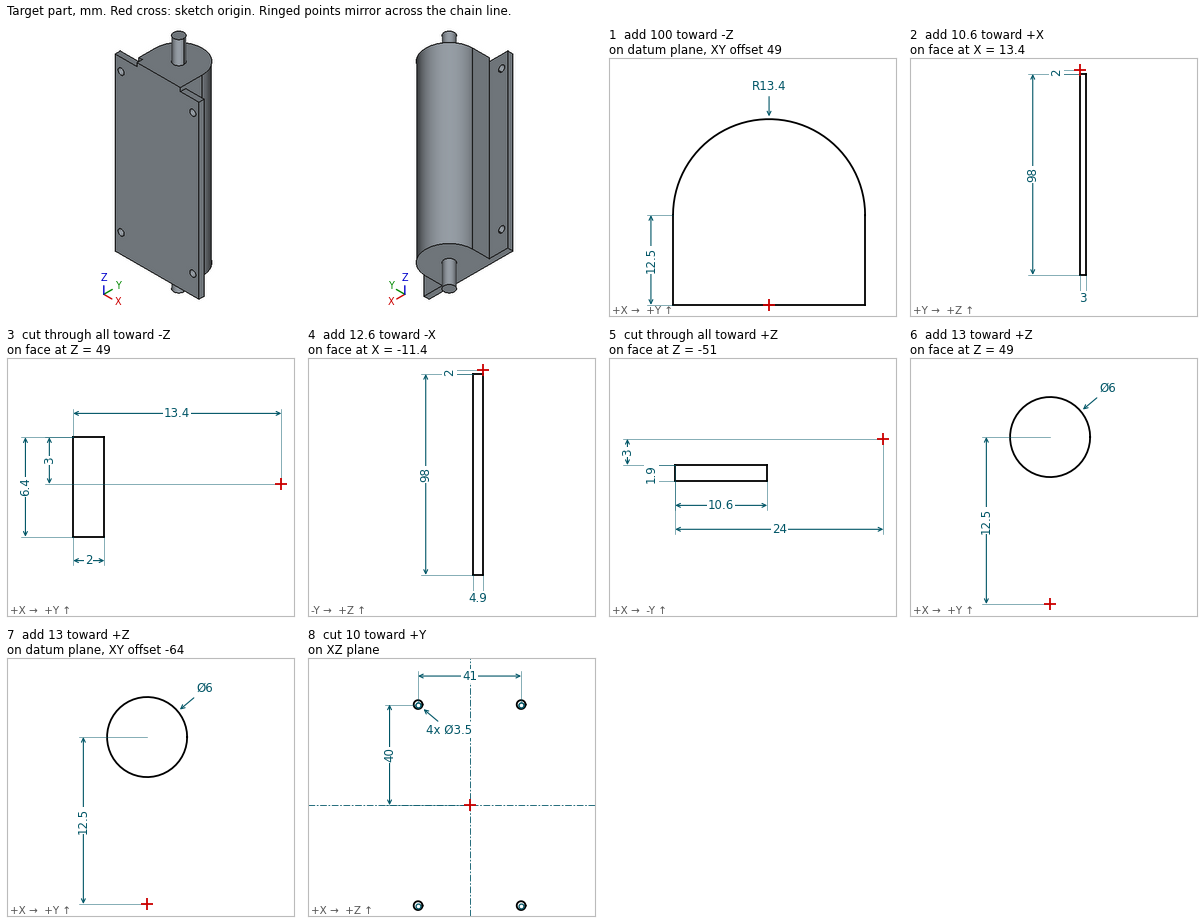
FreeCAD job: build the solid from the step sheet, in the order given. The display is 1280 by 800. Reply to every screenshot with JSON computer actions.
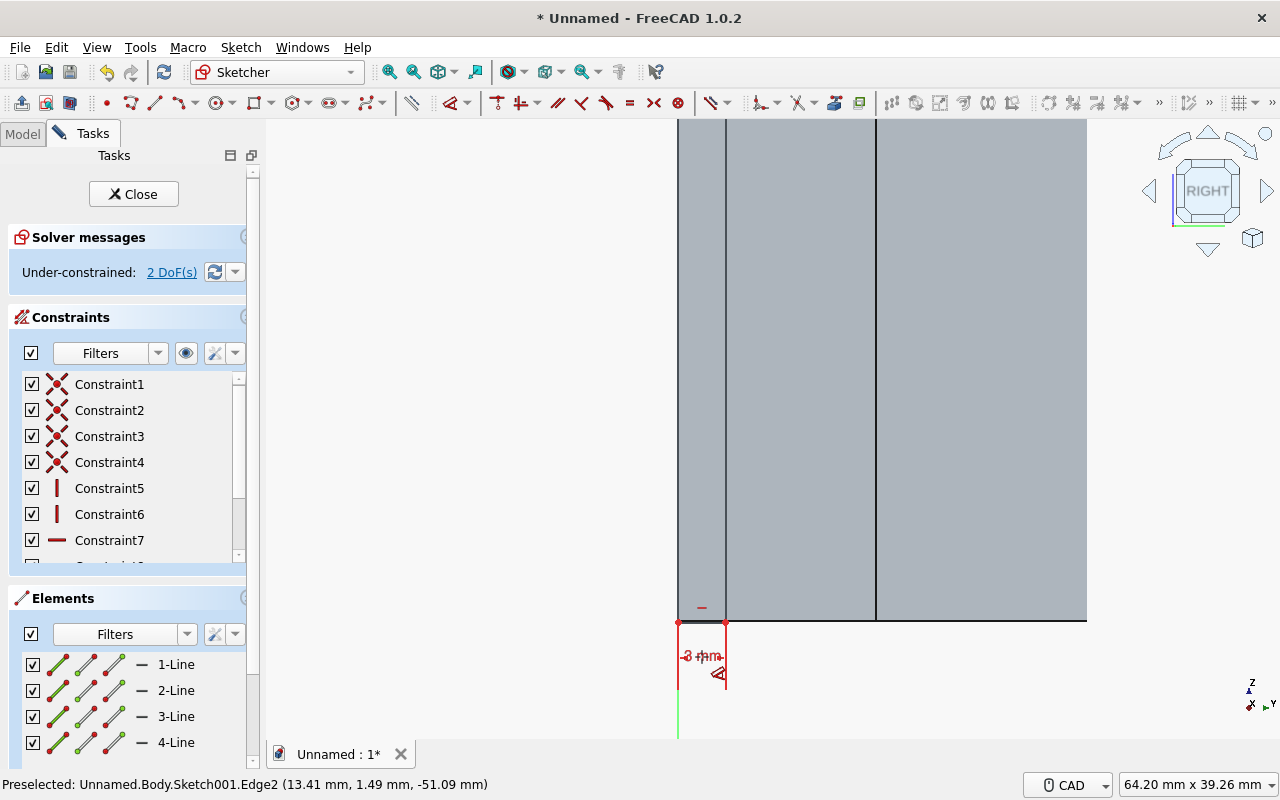
{"action": "scroll", "coordinate": [705, 625], "scroll_direction": "down", "scroll_amount": 7}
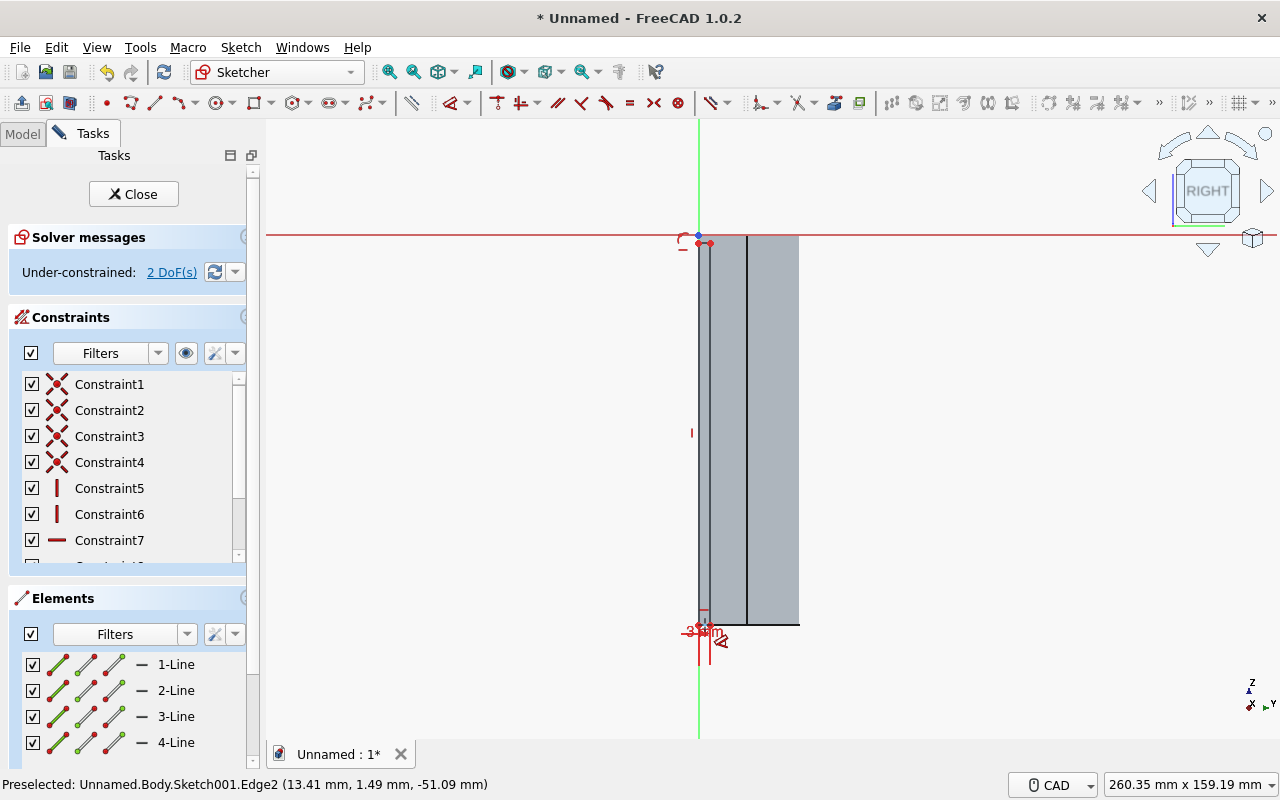
{"action": "left_click", "coordinate": [699, 511]}
{"action": "left_click", "coordinate": [665, 434]}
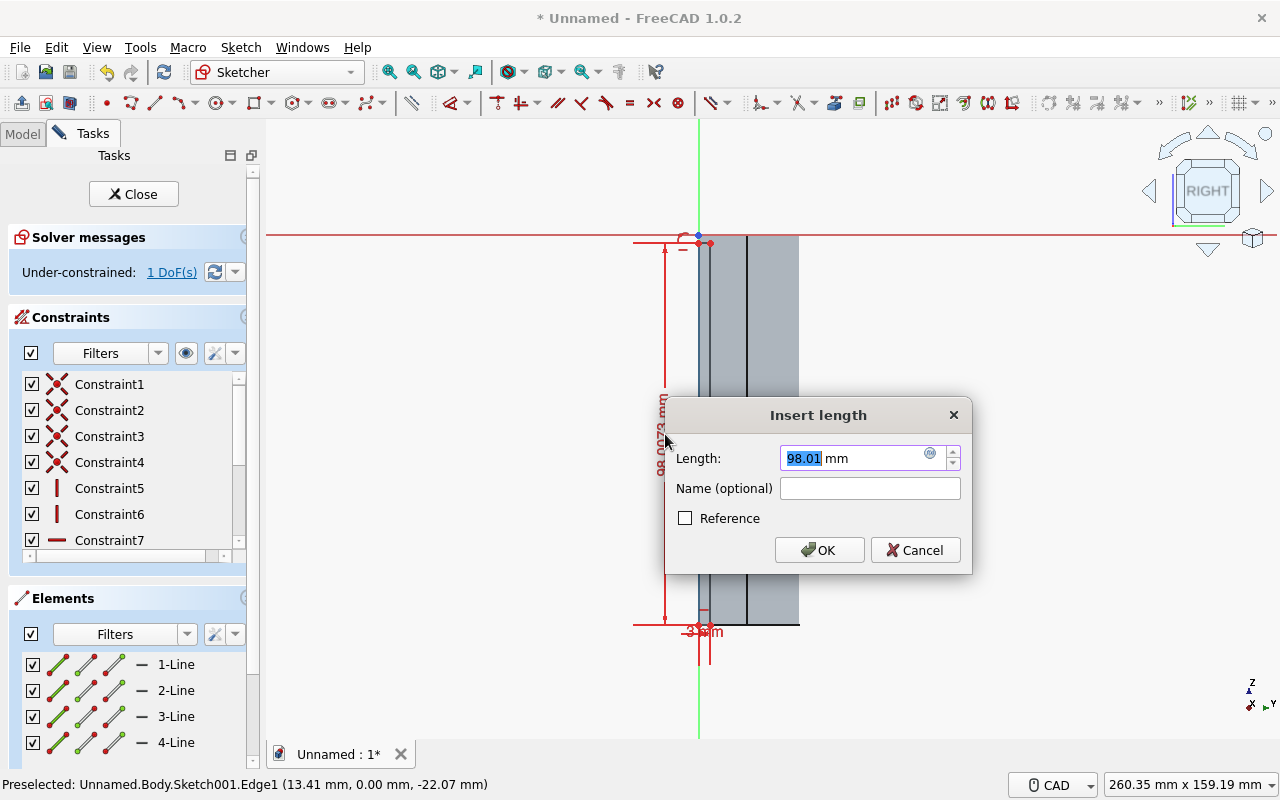
{"action": "type", "text": "98"}
{"action": "key", "text": "Return"}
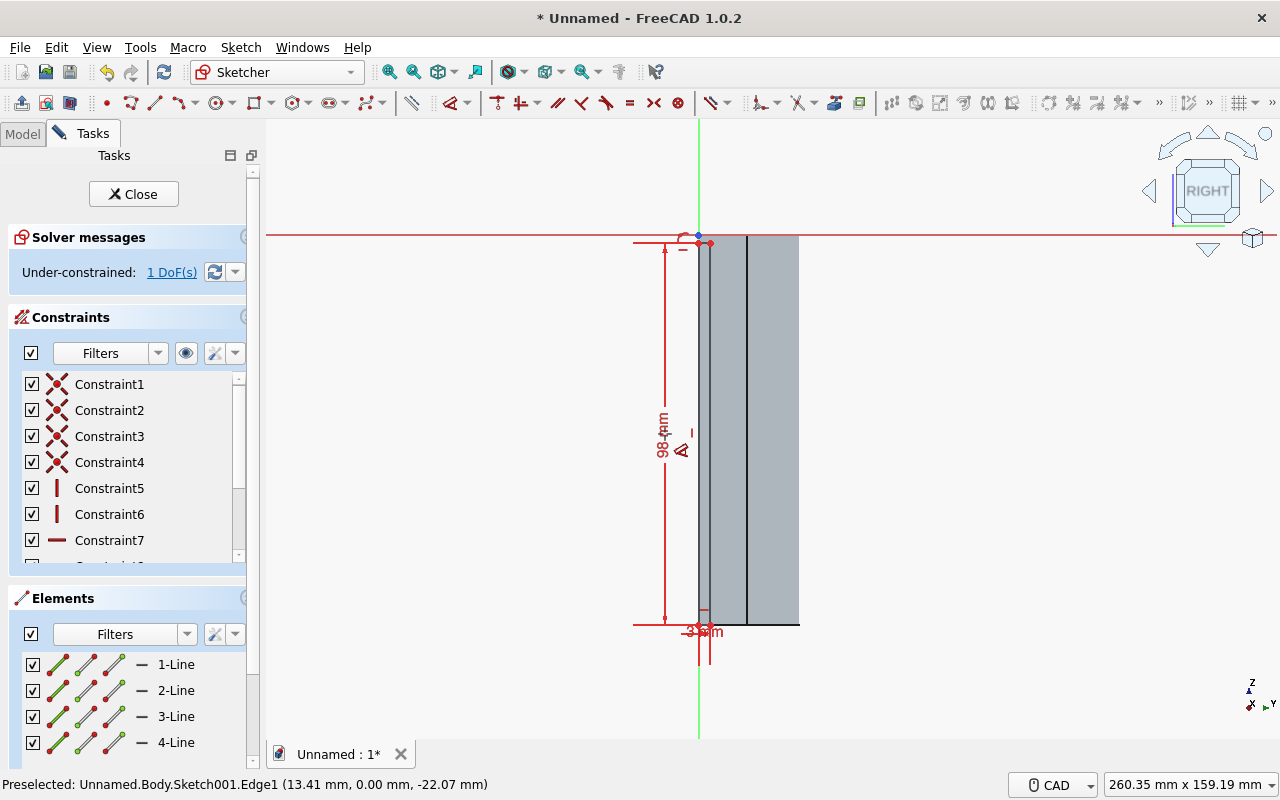
{"action": "scroll", "coordinate": [699, 243], "scroll_direction": "up", "scroll_amount": 9}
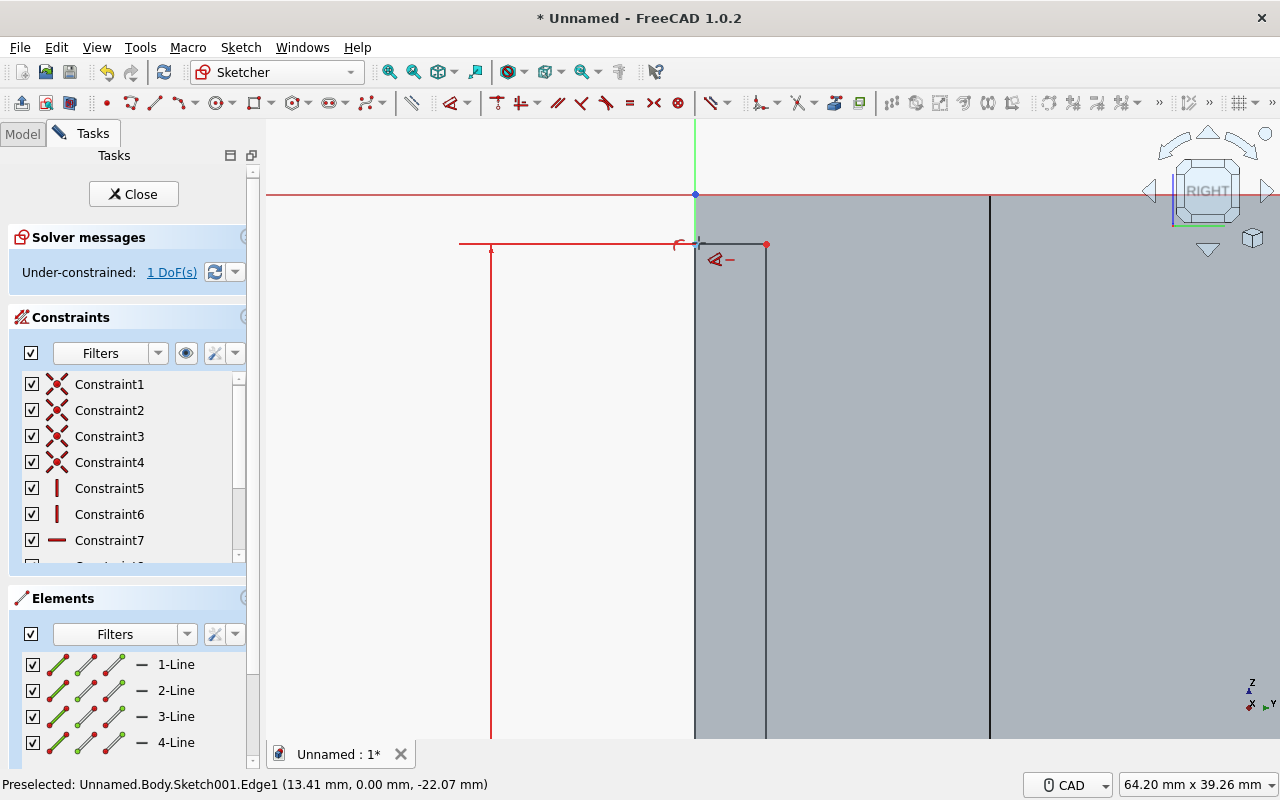
{"action": "left_click", "coordinate": [695, 244]}
{"action": "left_click", "coordinate": [661, 219]}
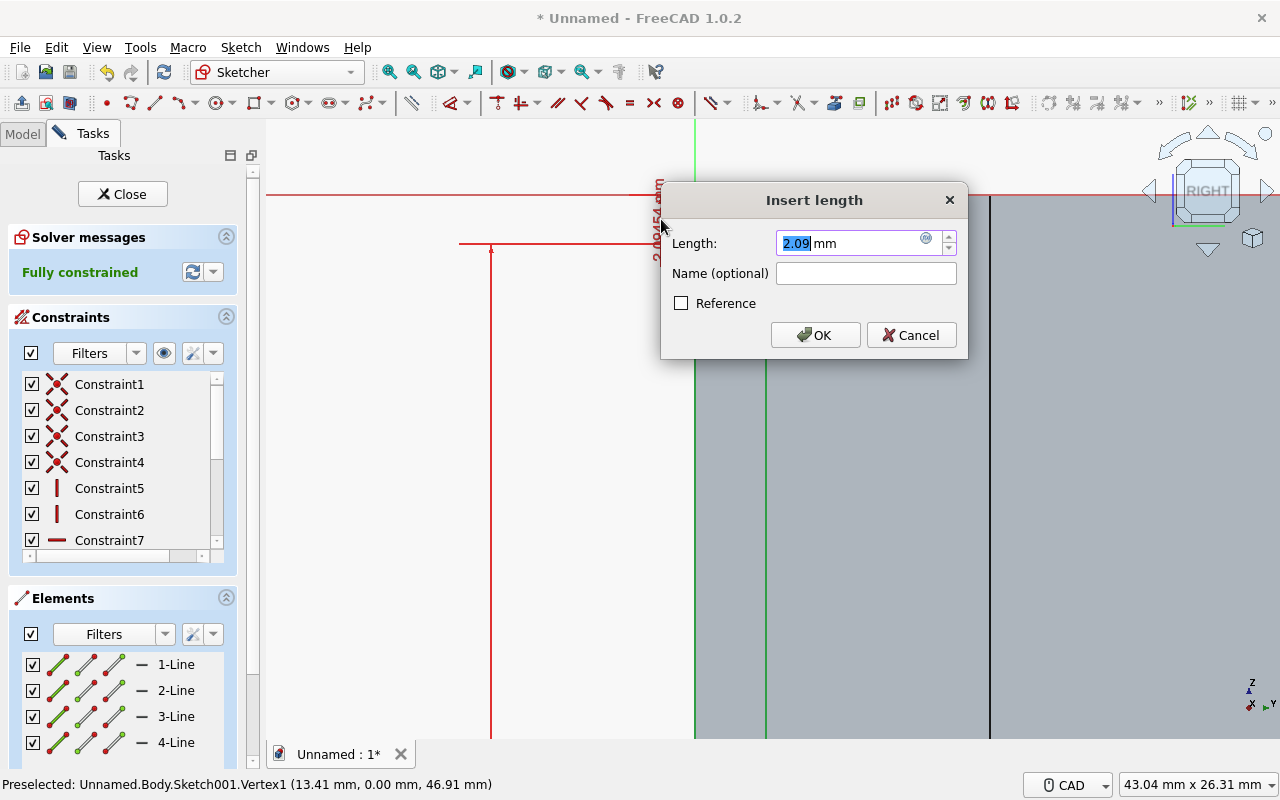
{"action": "type", "text": "2"}
{"action": "key", "text": "Return"}
{"action": "key", "text": "Escape"}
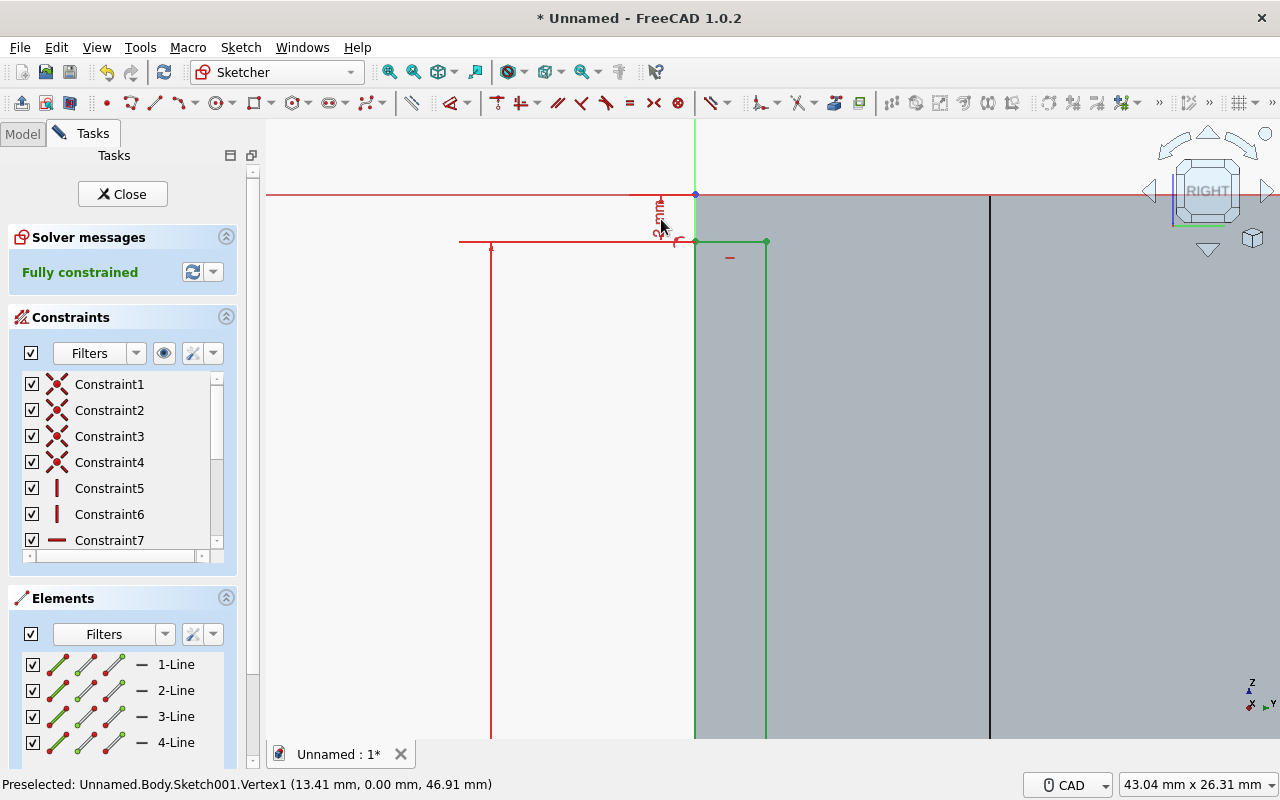
{"action": "left_click", "coordinate": [123, 194]}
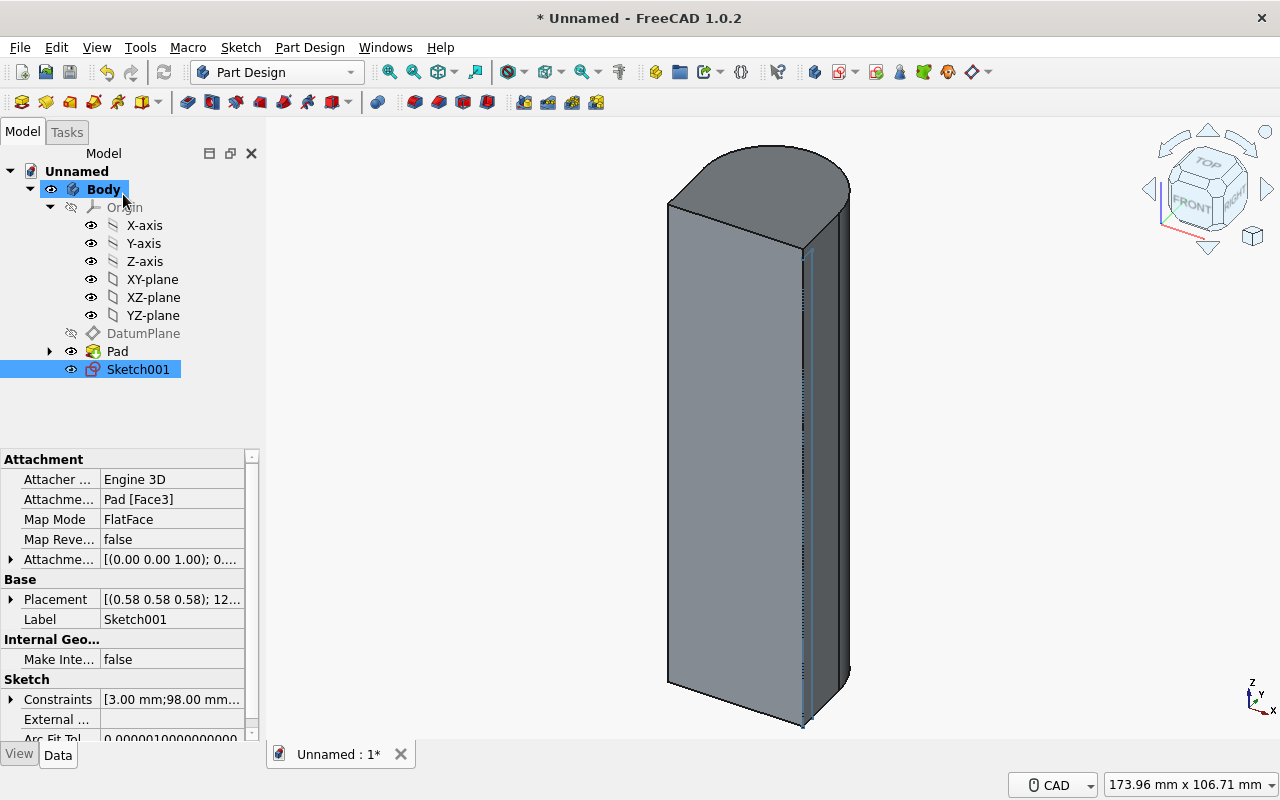
{"action": "left_click", "coordinate": [22, 102]}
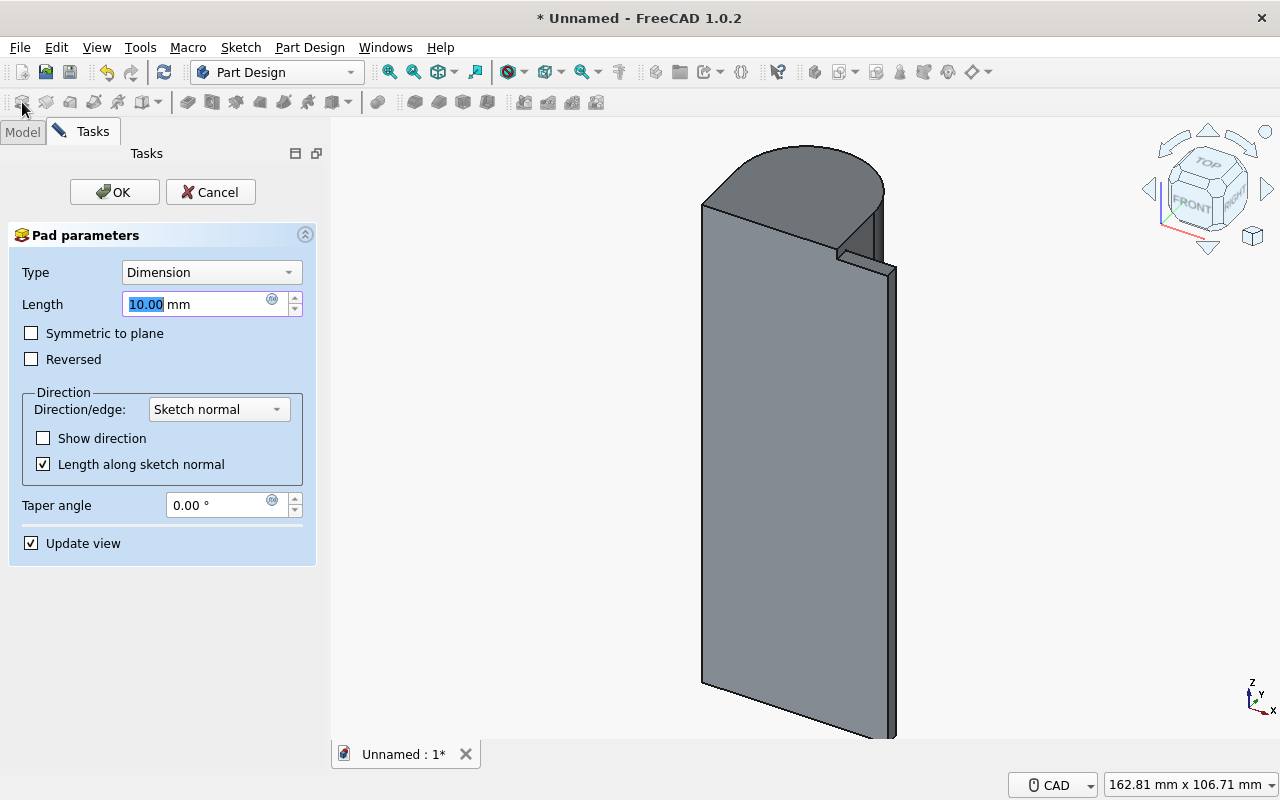
{"action": "type", "text": "10.6"}
{"action": "key", "text": "Tab"}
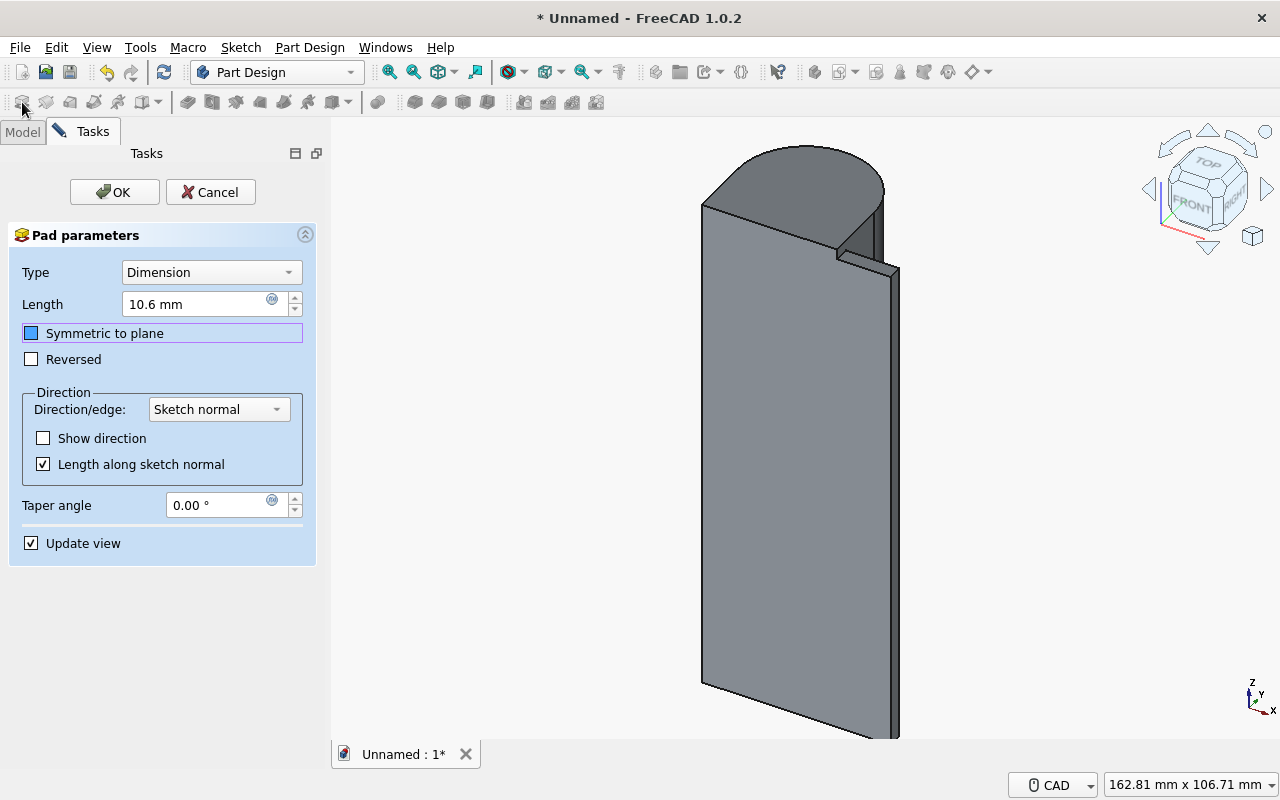
{"action": "left_click", "coordinate": [115, 192]}